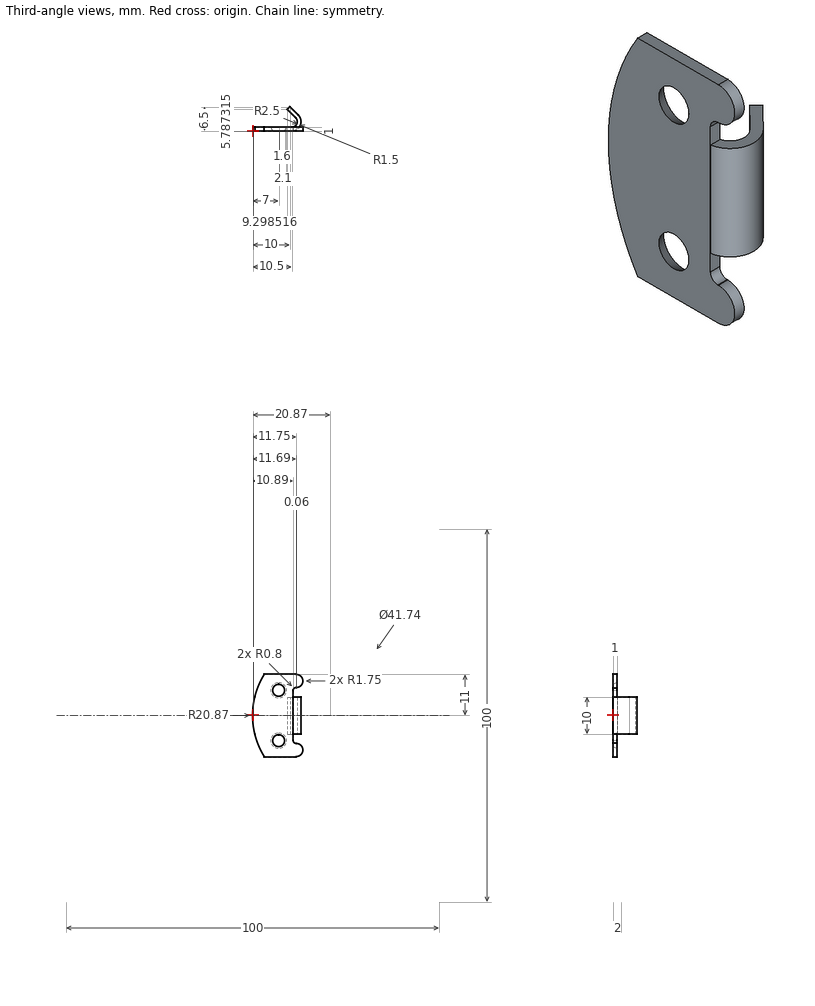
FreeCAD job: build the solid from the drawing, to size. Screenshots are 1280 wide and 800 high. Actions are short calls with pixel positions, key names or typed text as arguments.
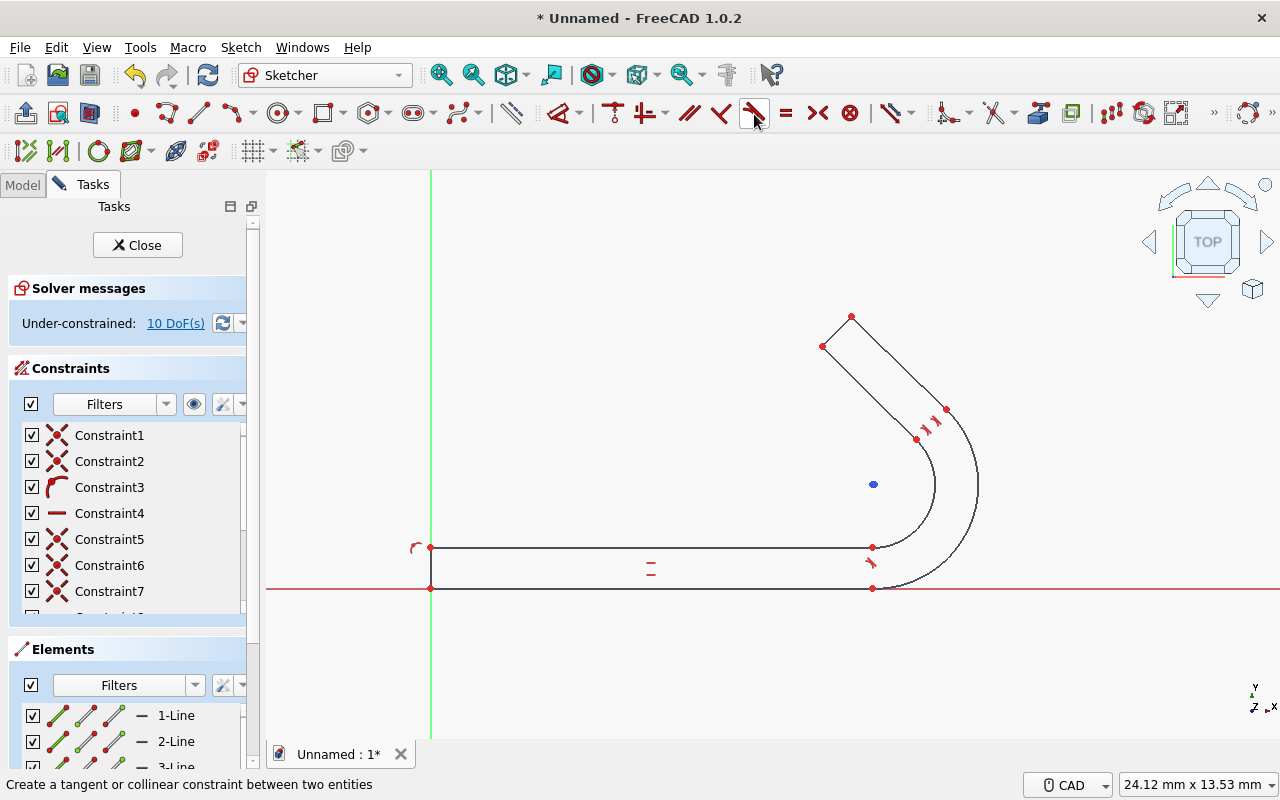
click(563, 589)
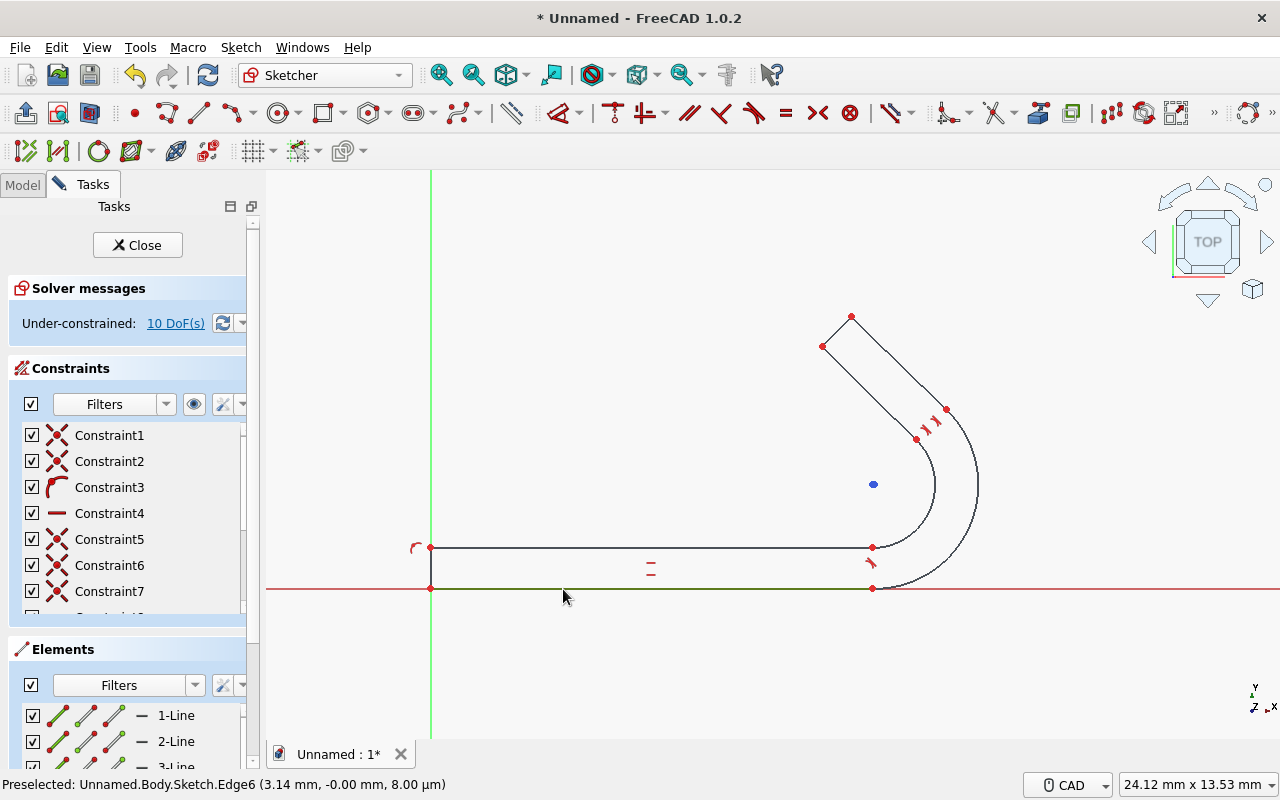
click(941, 565)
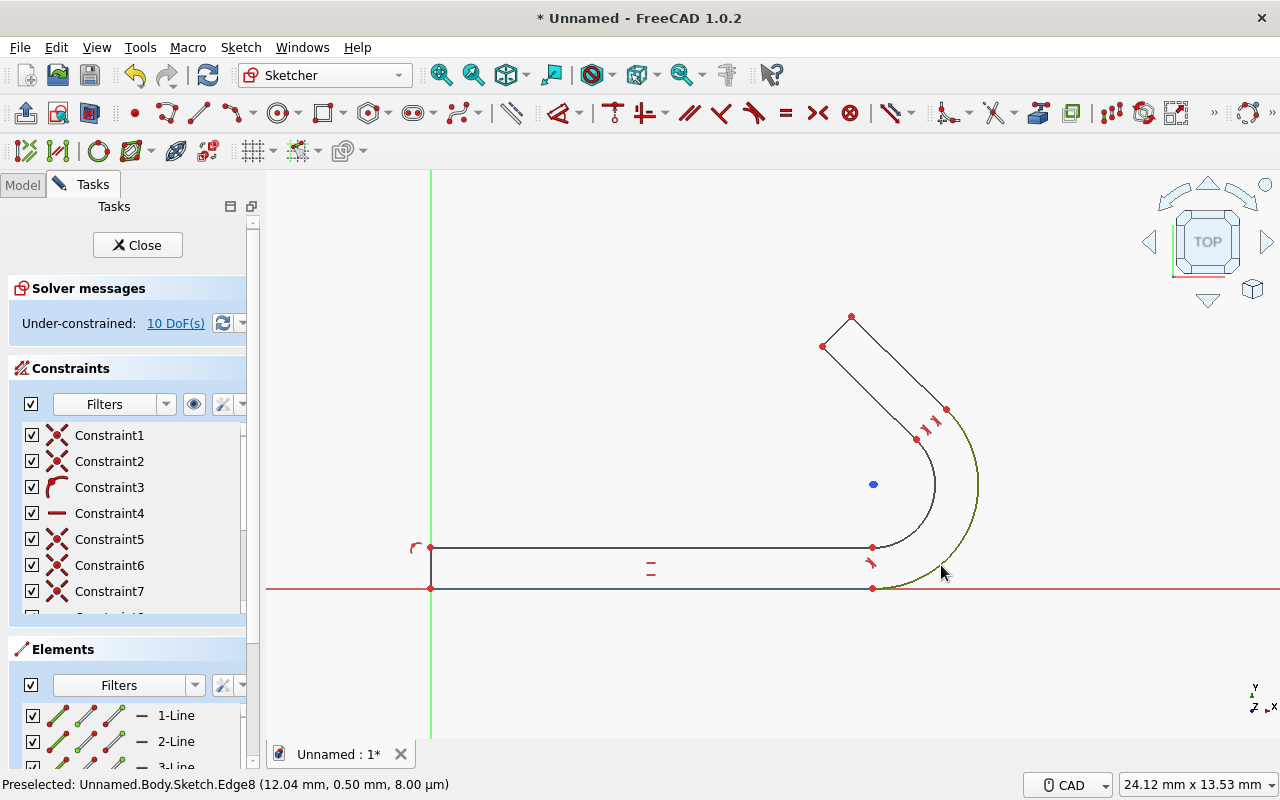
click(754, 114)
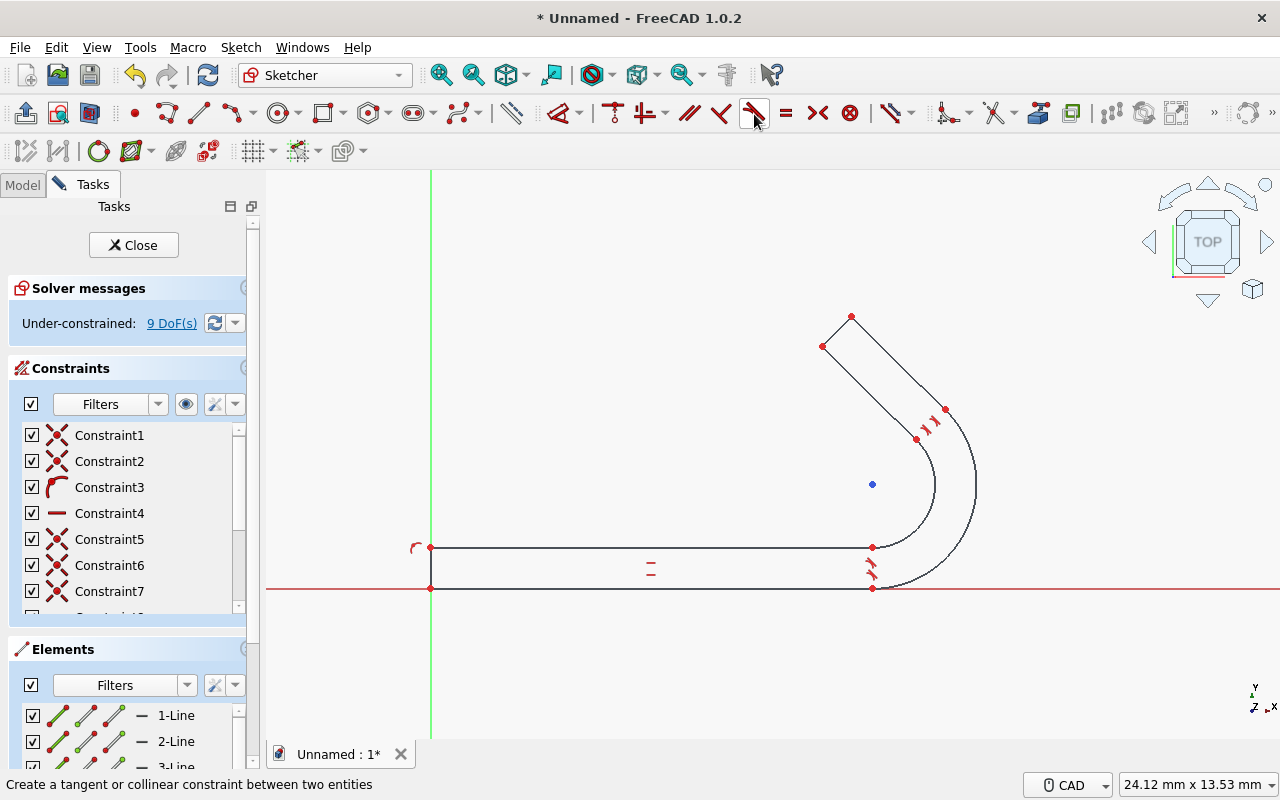
click(913, 533)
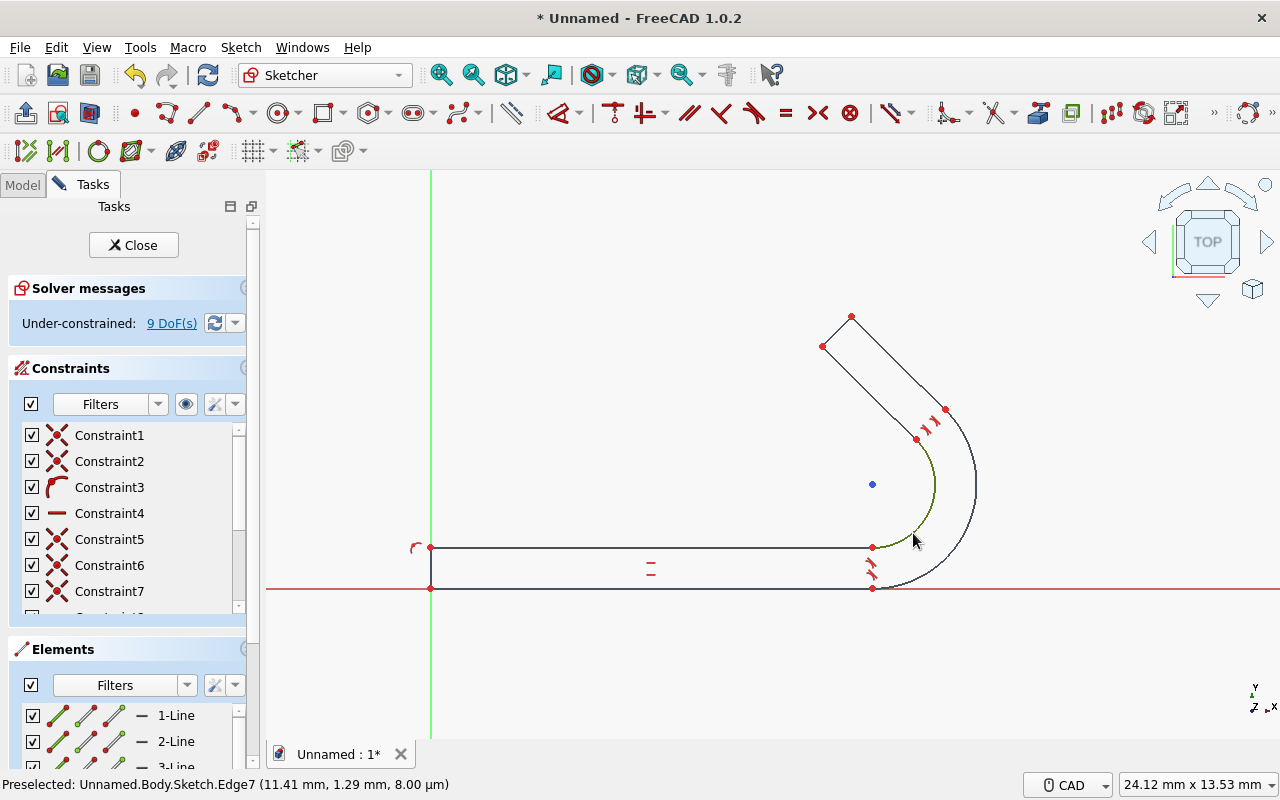
click(940, 564)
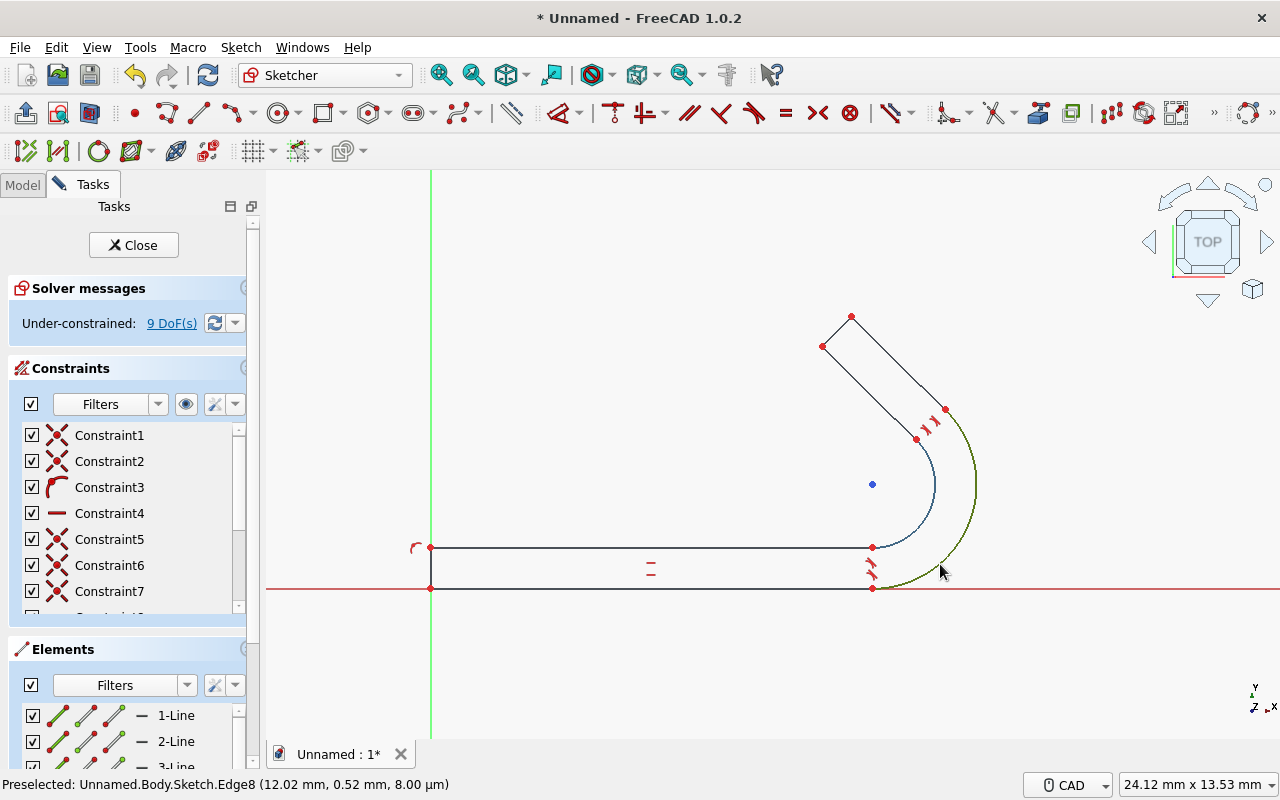
key(c)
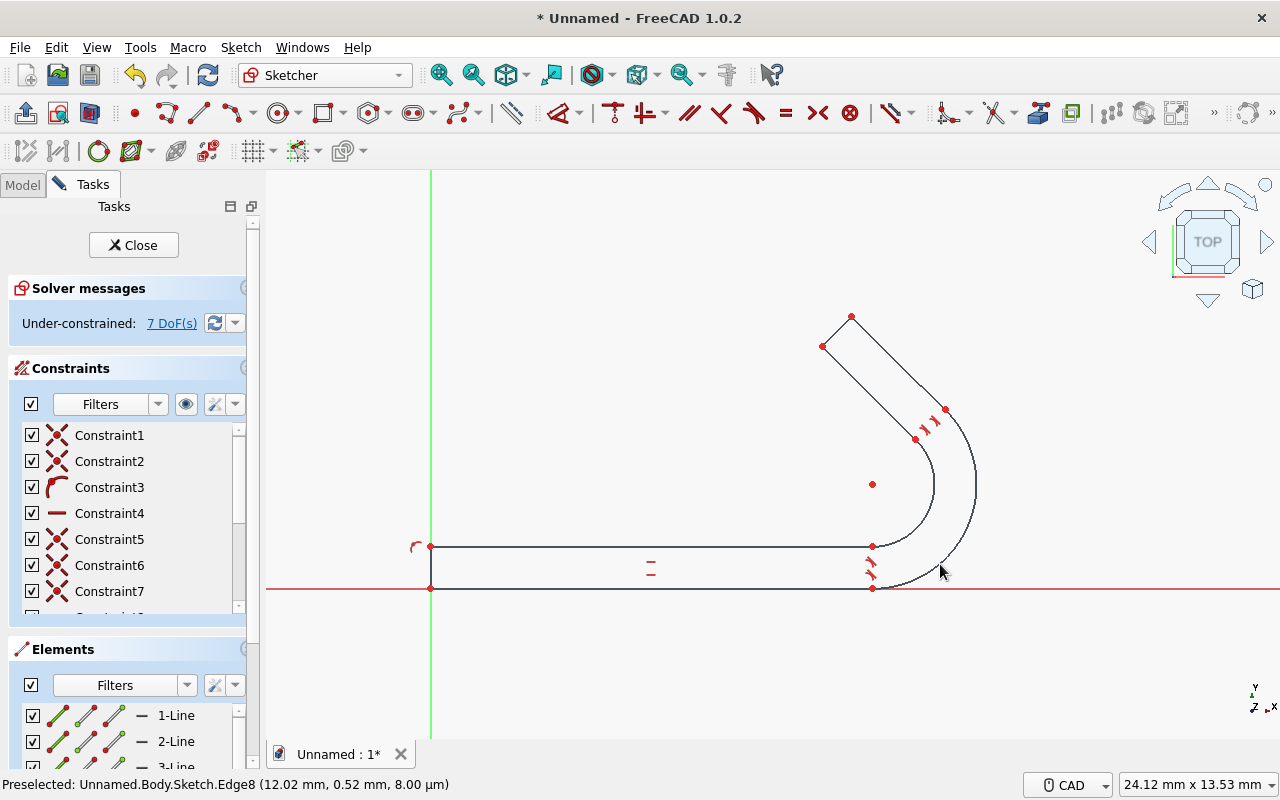
click(558, 114)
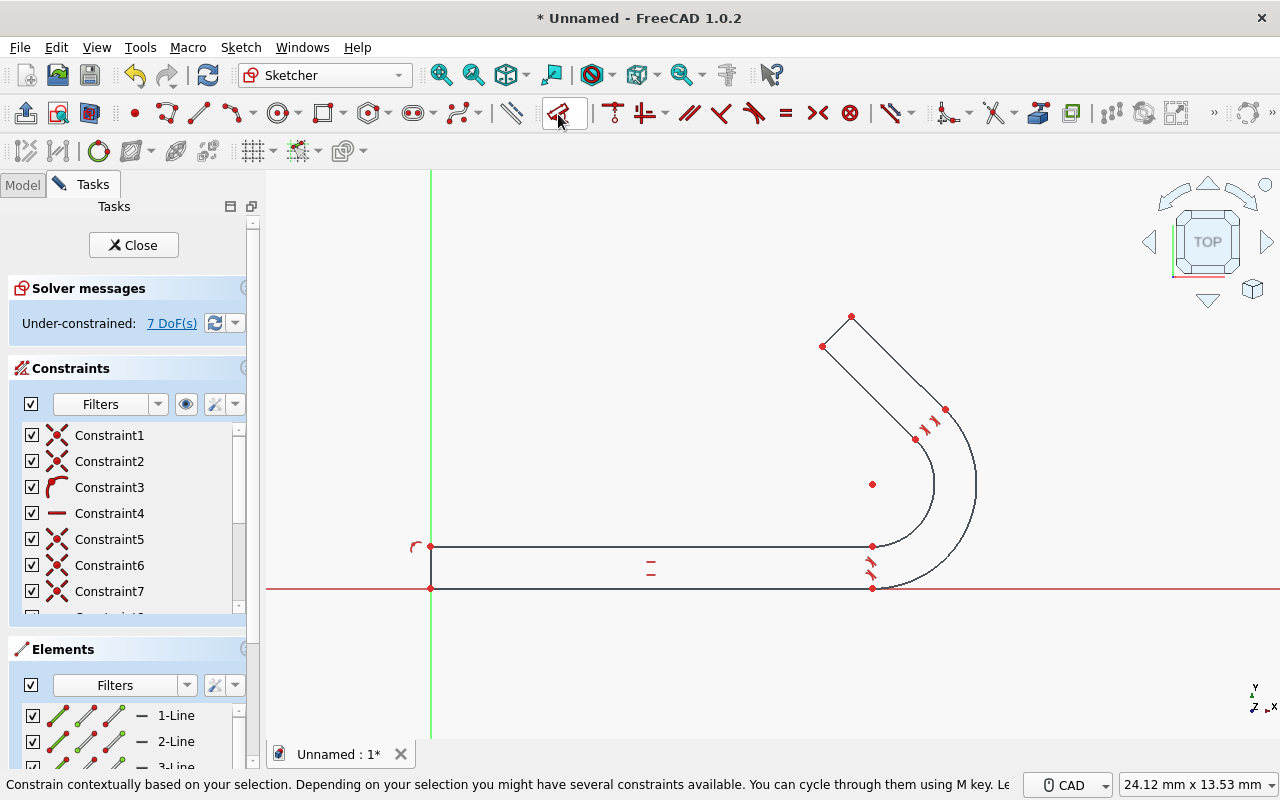
click(913, 532)
click(845, 575)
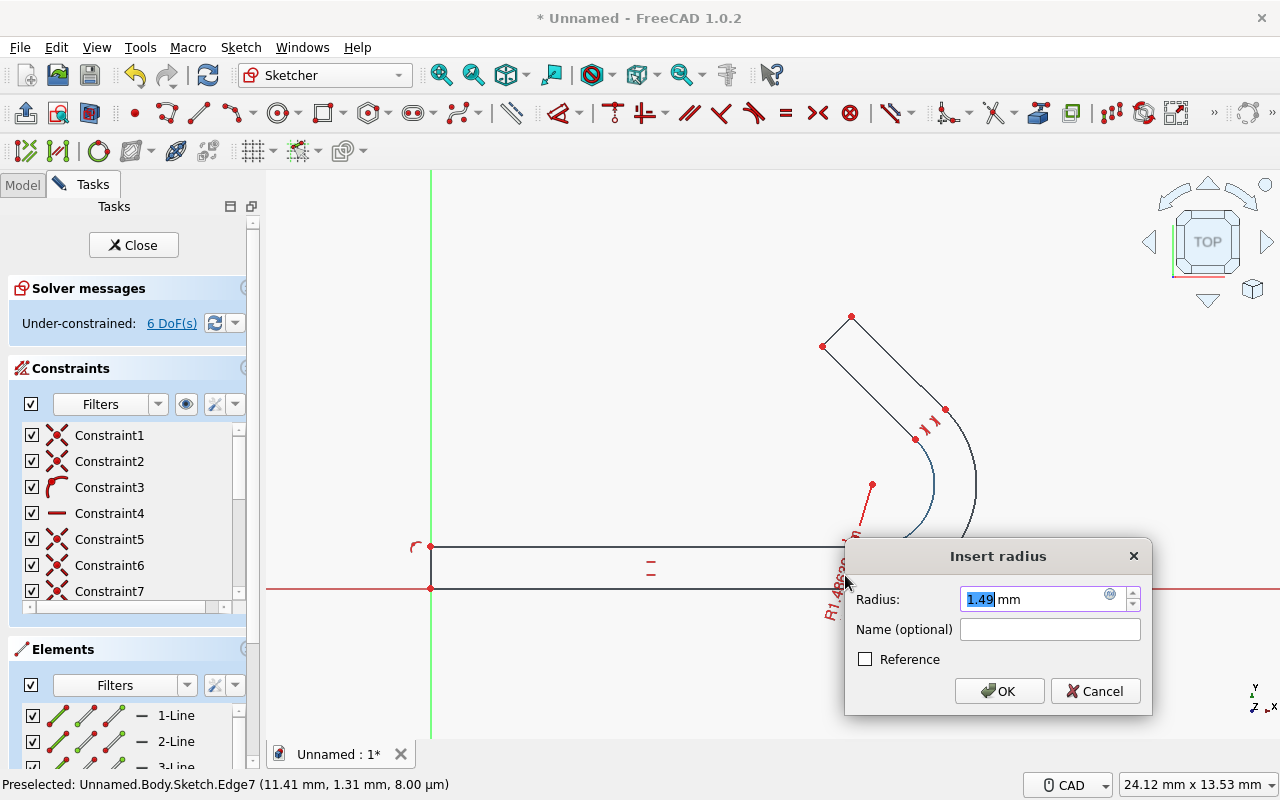
text(1.5)
key(Return)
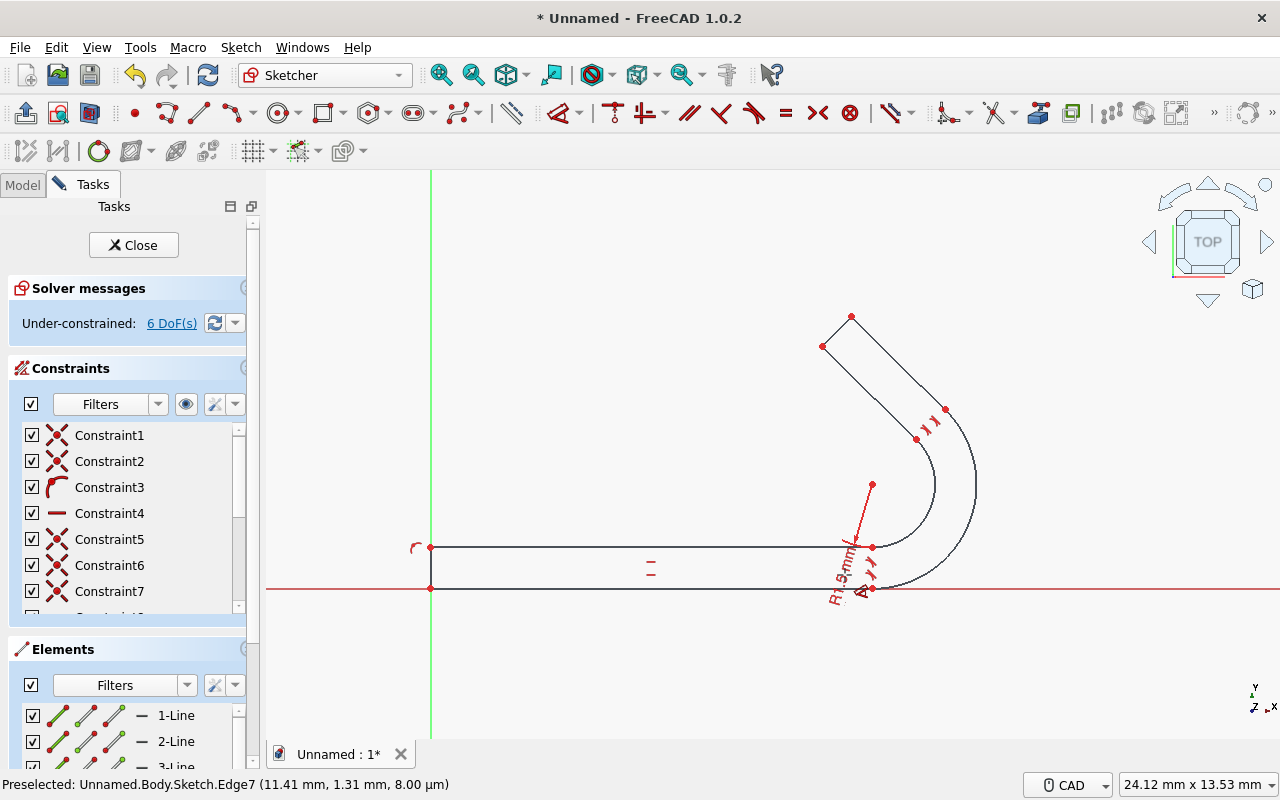
click(940, 564)
click(900, 618)